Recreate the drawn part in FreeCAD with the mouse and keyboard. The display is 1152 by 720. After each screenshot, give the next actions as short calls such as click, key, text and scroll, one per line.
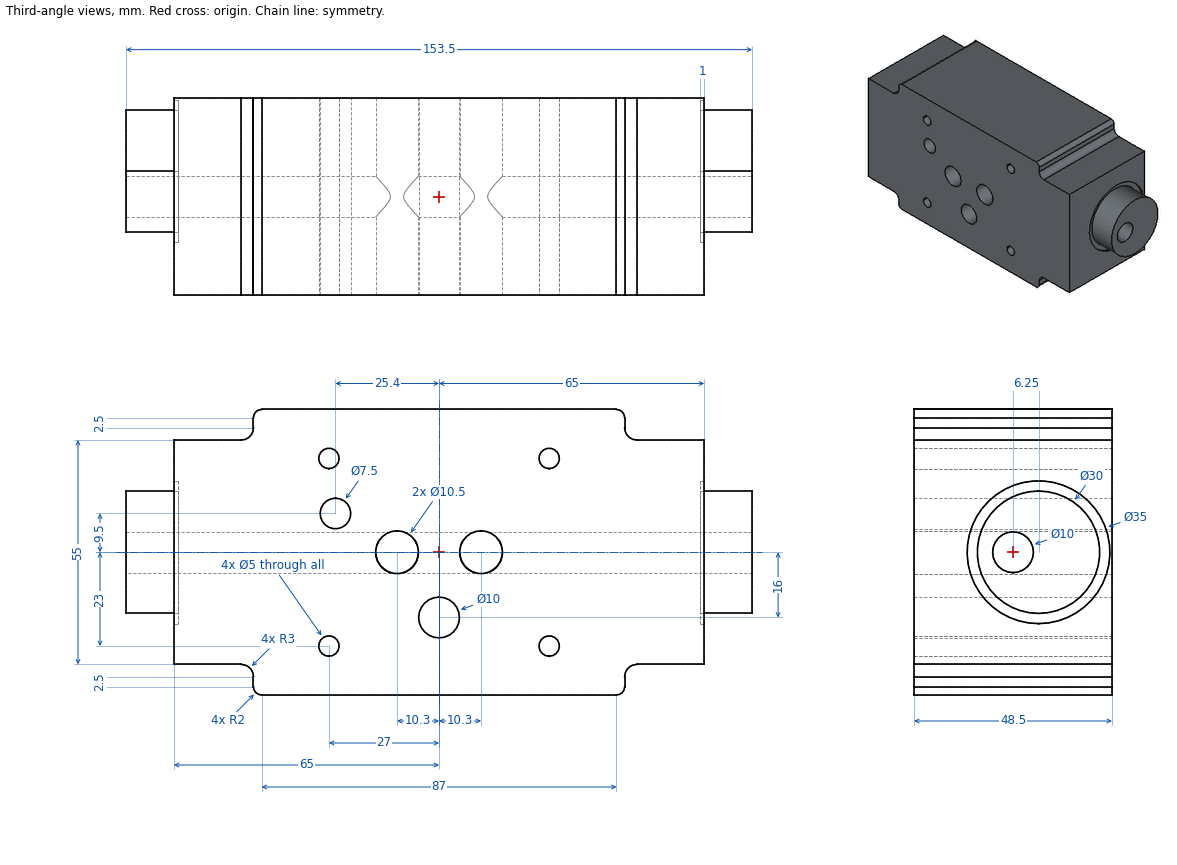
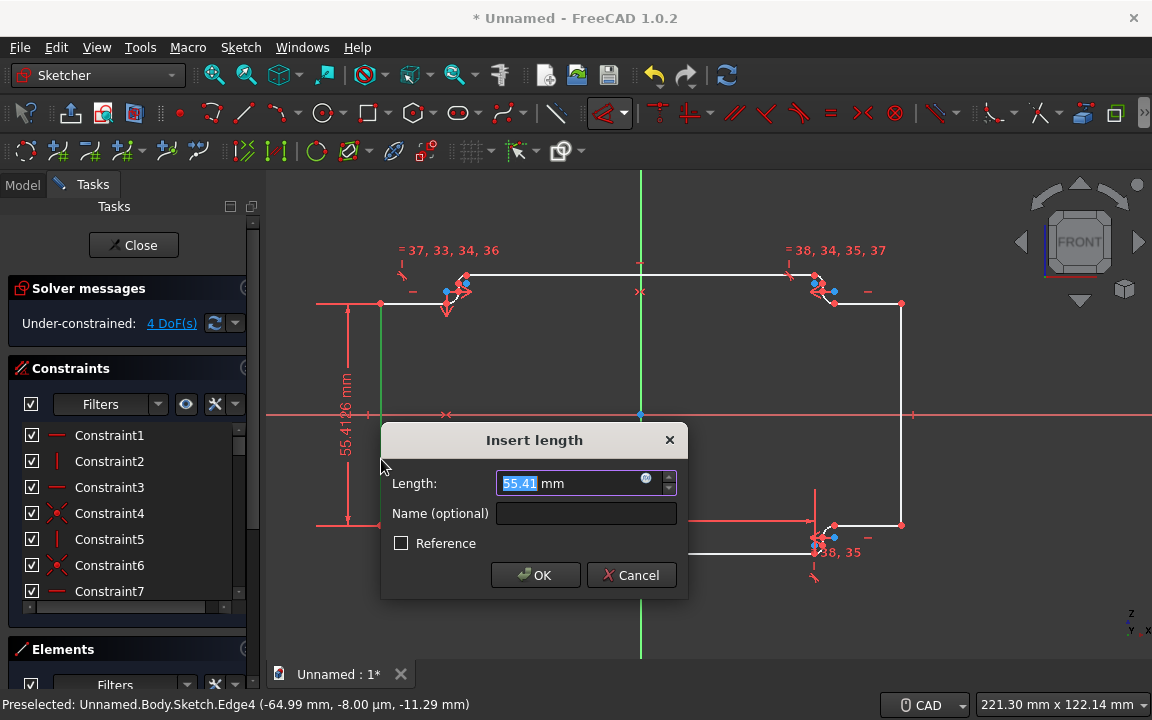
text(55)
key(Return)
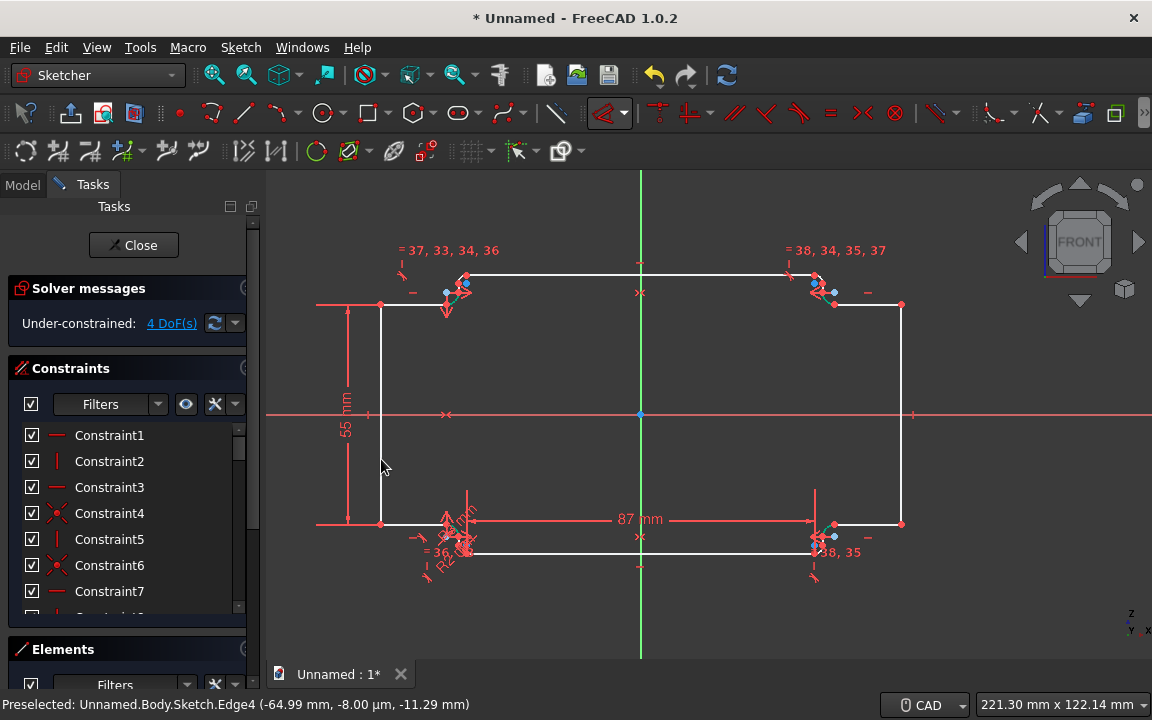
scroll(459, 541, up, 7)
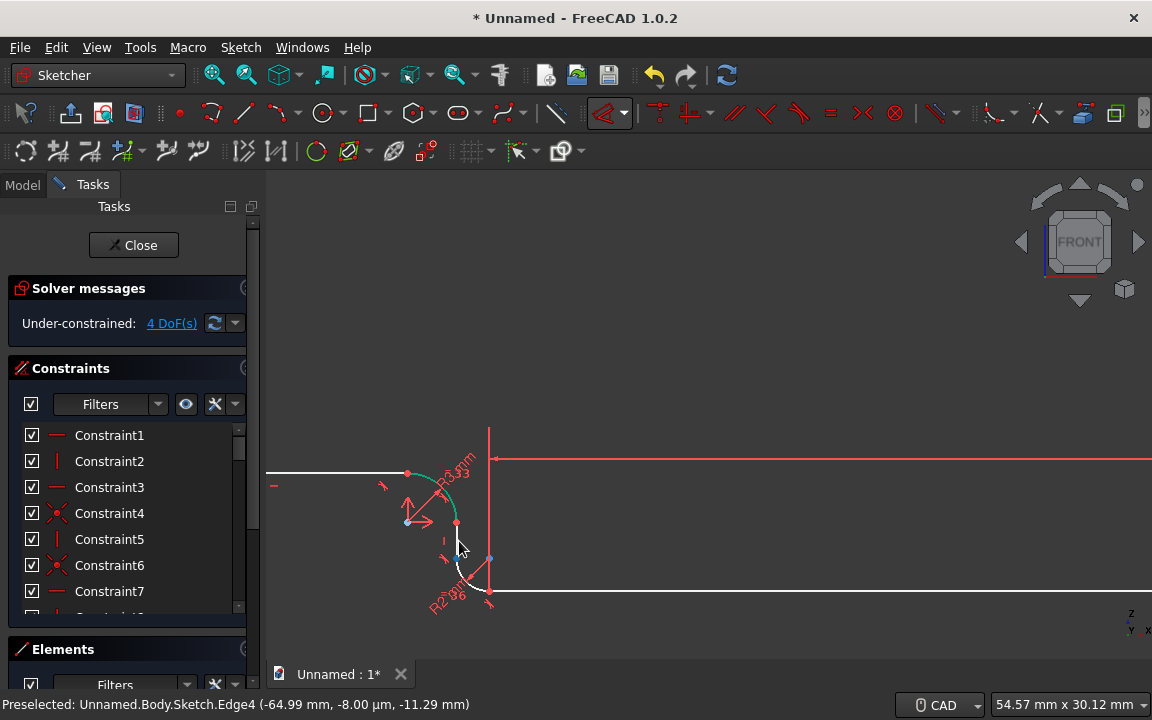
click(457, 540)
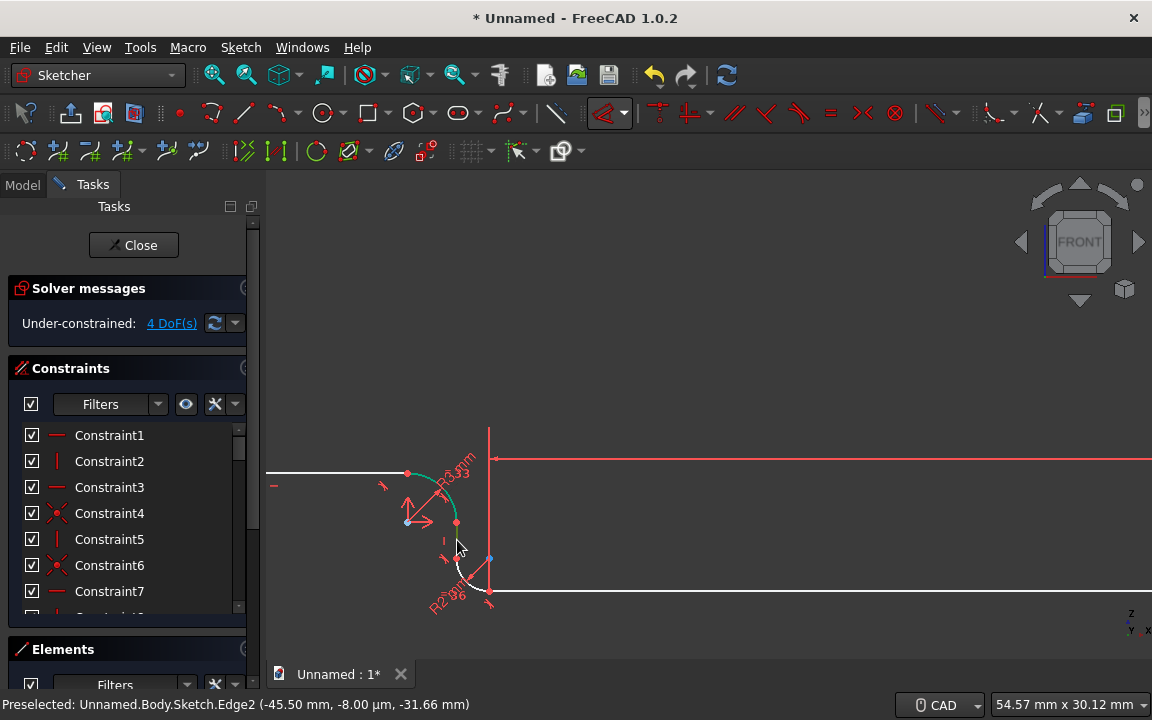
click(626, 114)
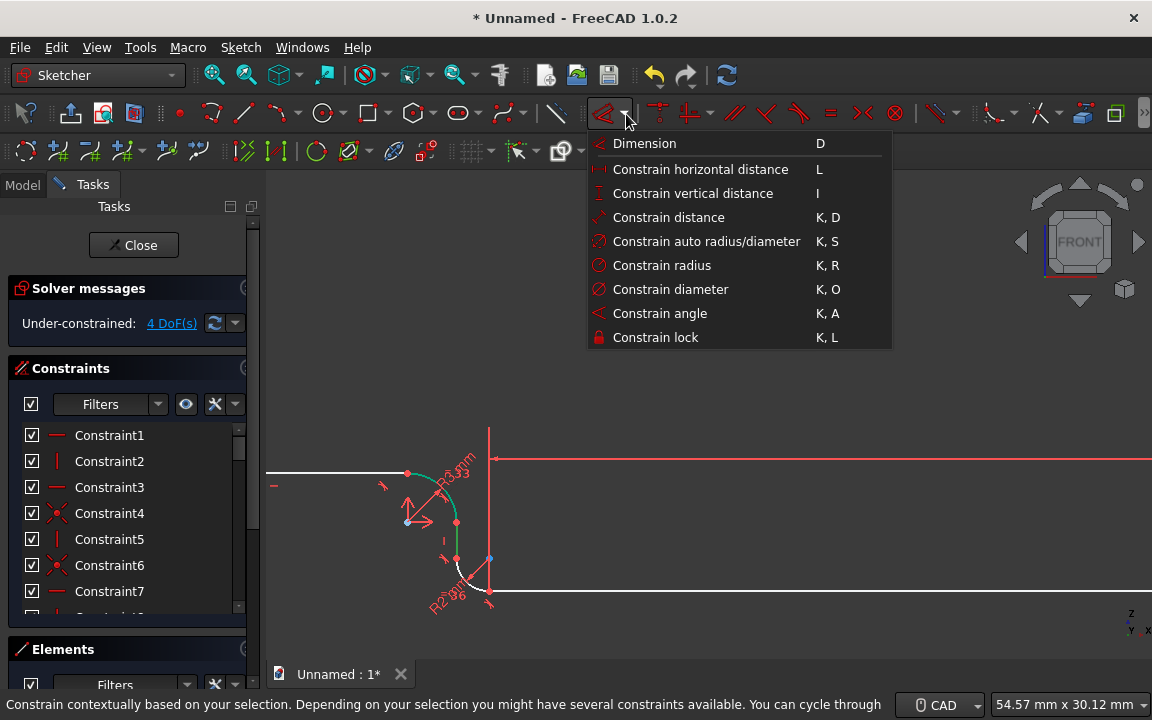
click(740, 193)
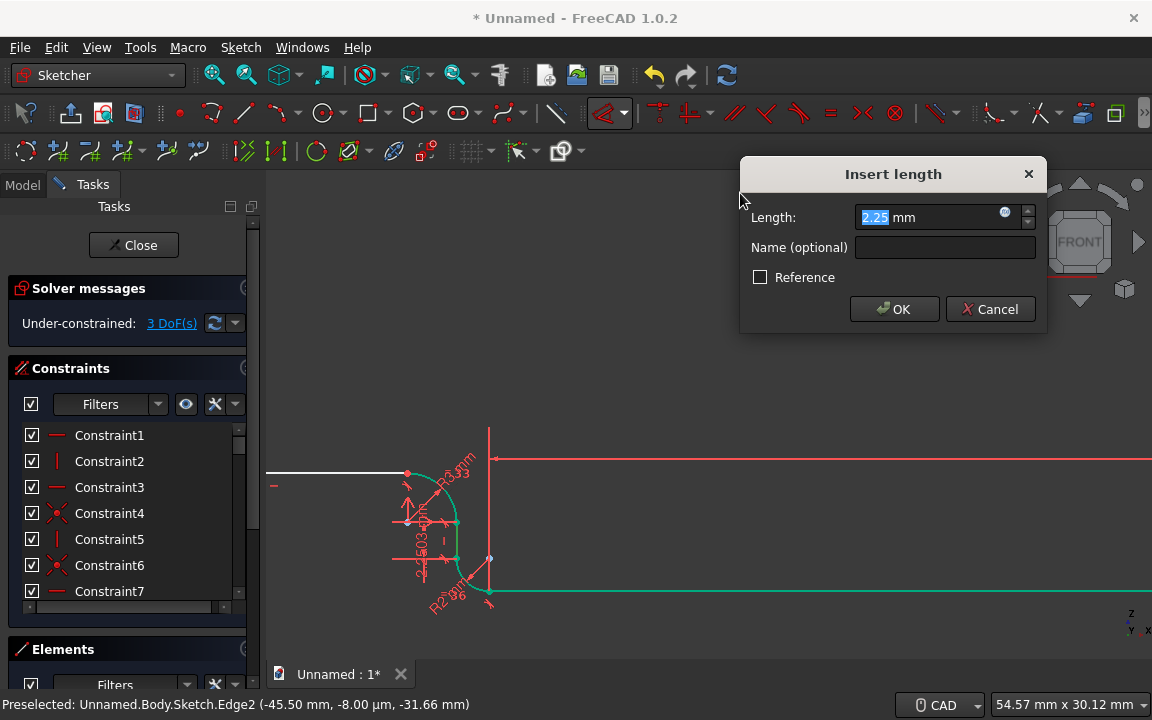
text(2.5)
key(Return)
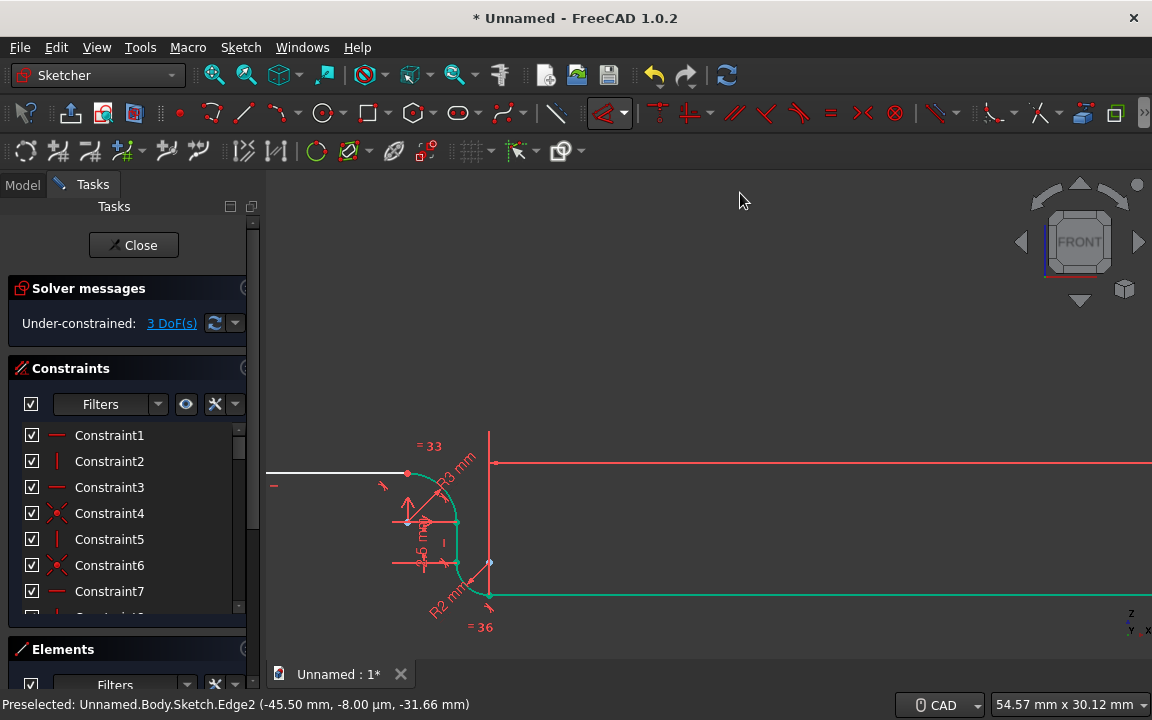
scroll(459, 541, down, 7)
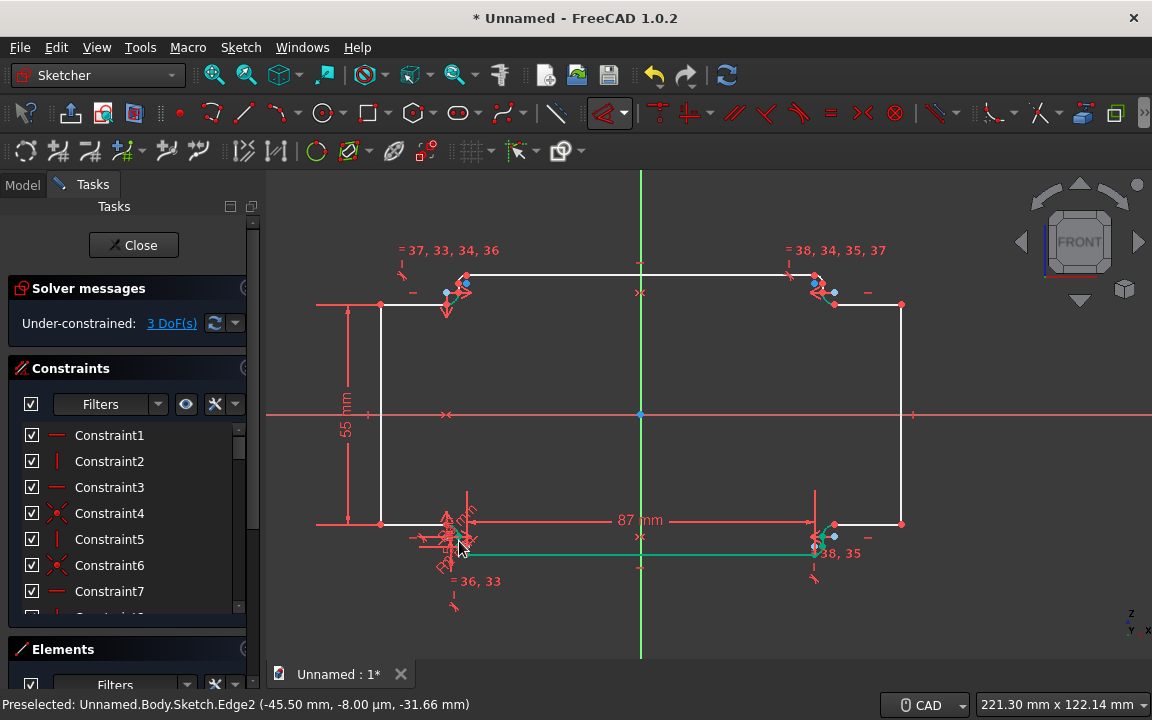
scroll(459, 290, up, 8)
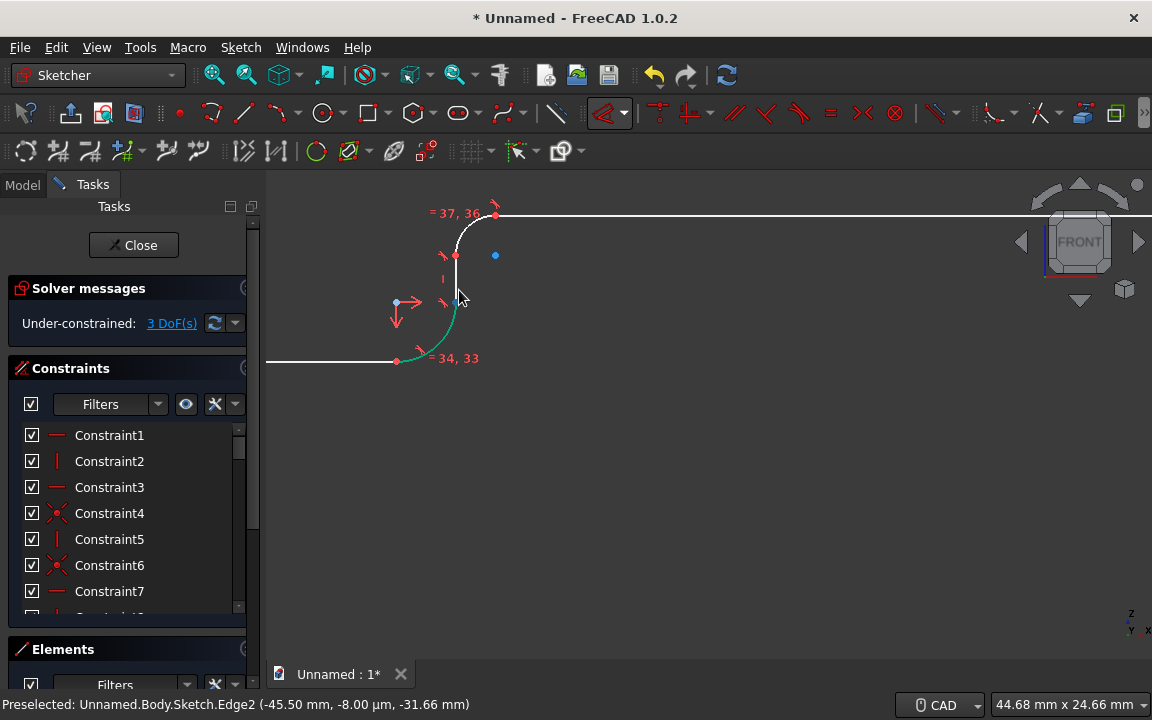
click(456, 288)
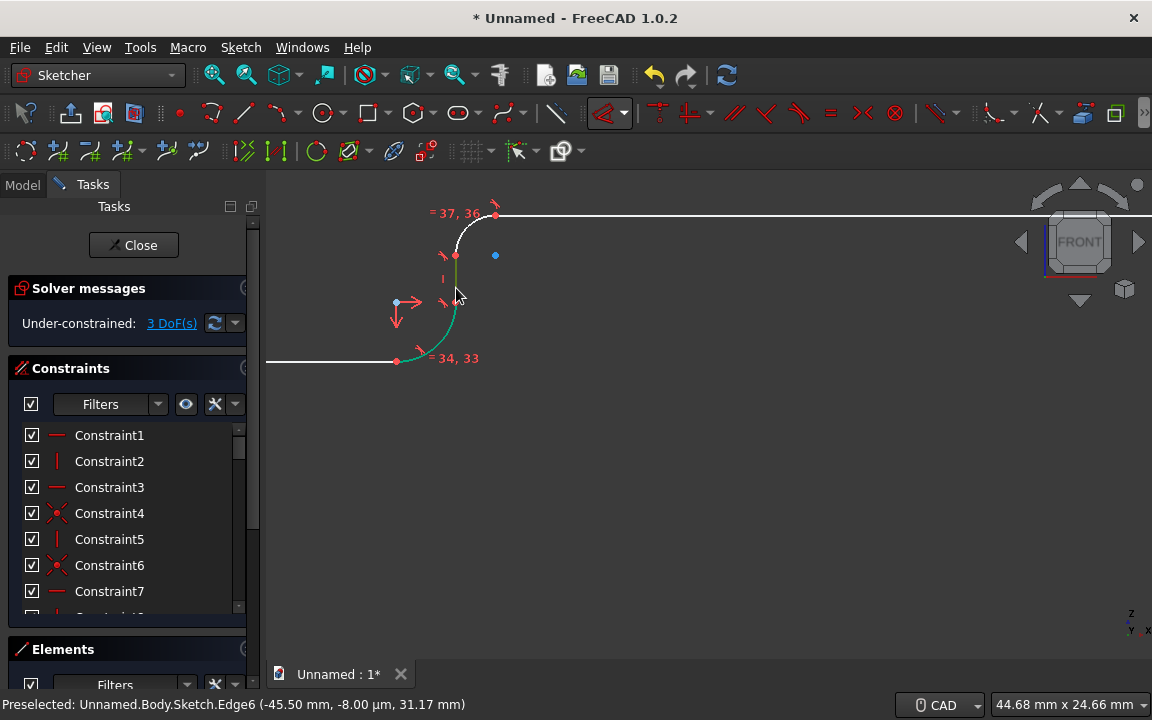
key(i)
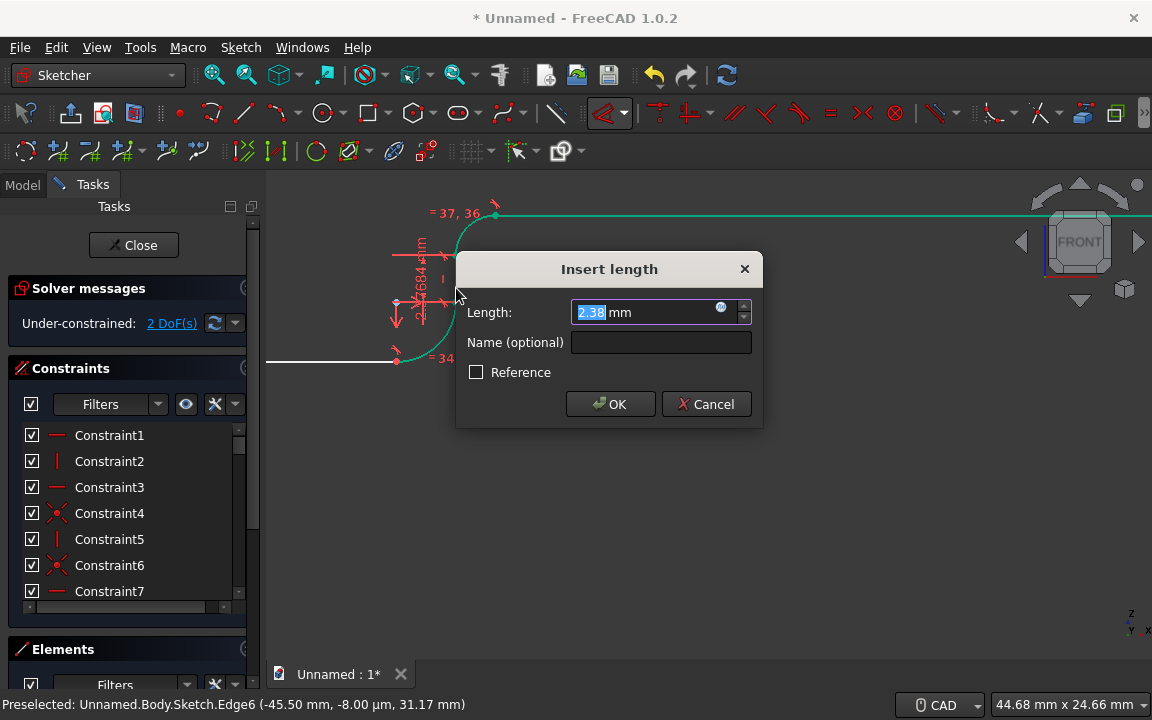
text(2.5)
key(Return)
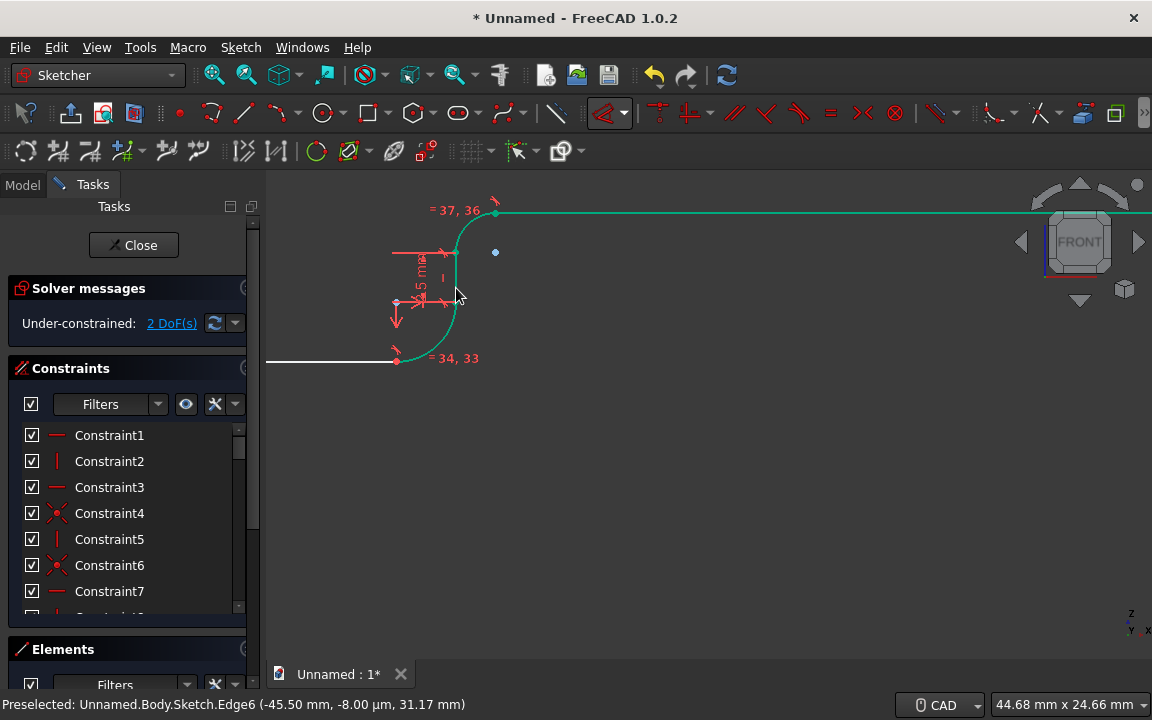
scroll(459, 290, down, 8)